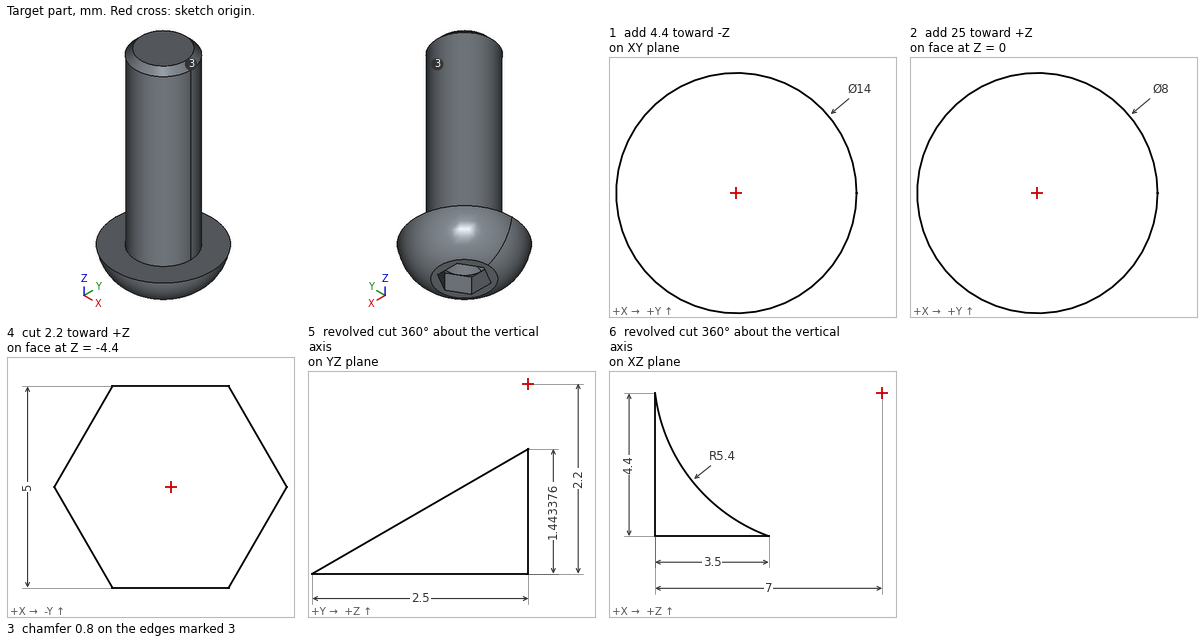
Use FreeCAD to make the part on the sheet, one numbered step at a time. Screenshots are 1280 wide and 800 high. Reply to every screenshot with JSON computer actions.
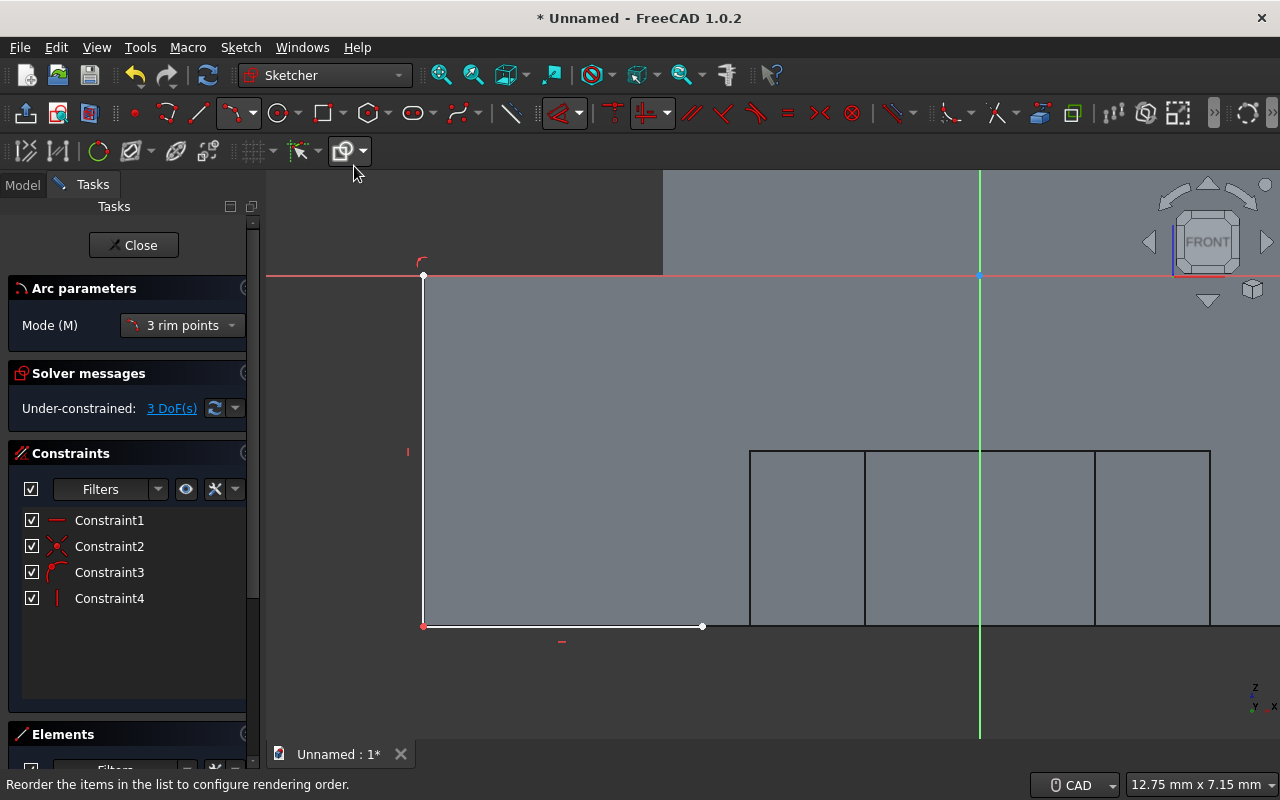
{"action": "left_click", "coordinate": [423, 276]}
{"action": "left_click", "coordinate": [702, 627]}
{"action": "left_click", "coordinate": [513, 490]}
{"action": "key", "text": "Escape"}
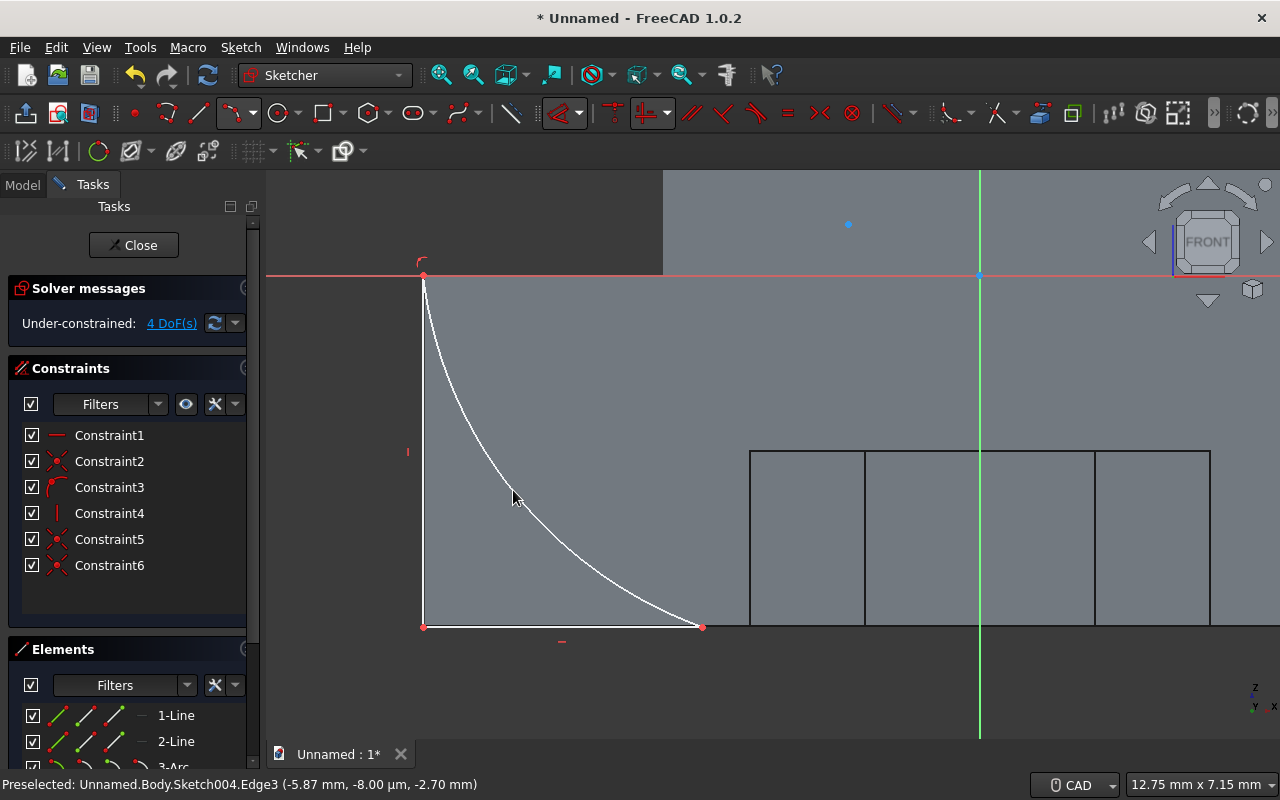
{"action": "left_click", "coordinate": [463, 411]}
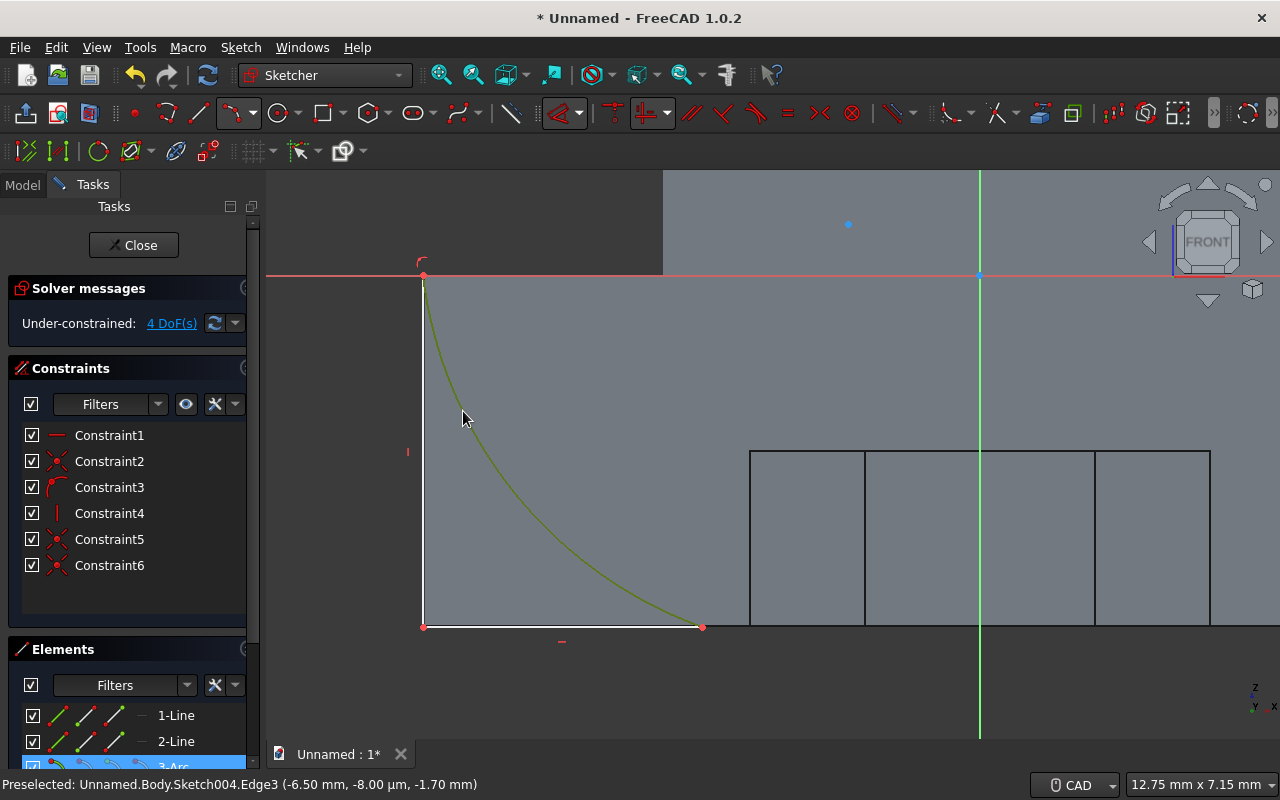
{"action": "key", "text": "k r"}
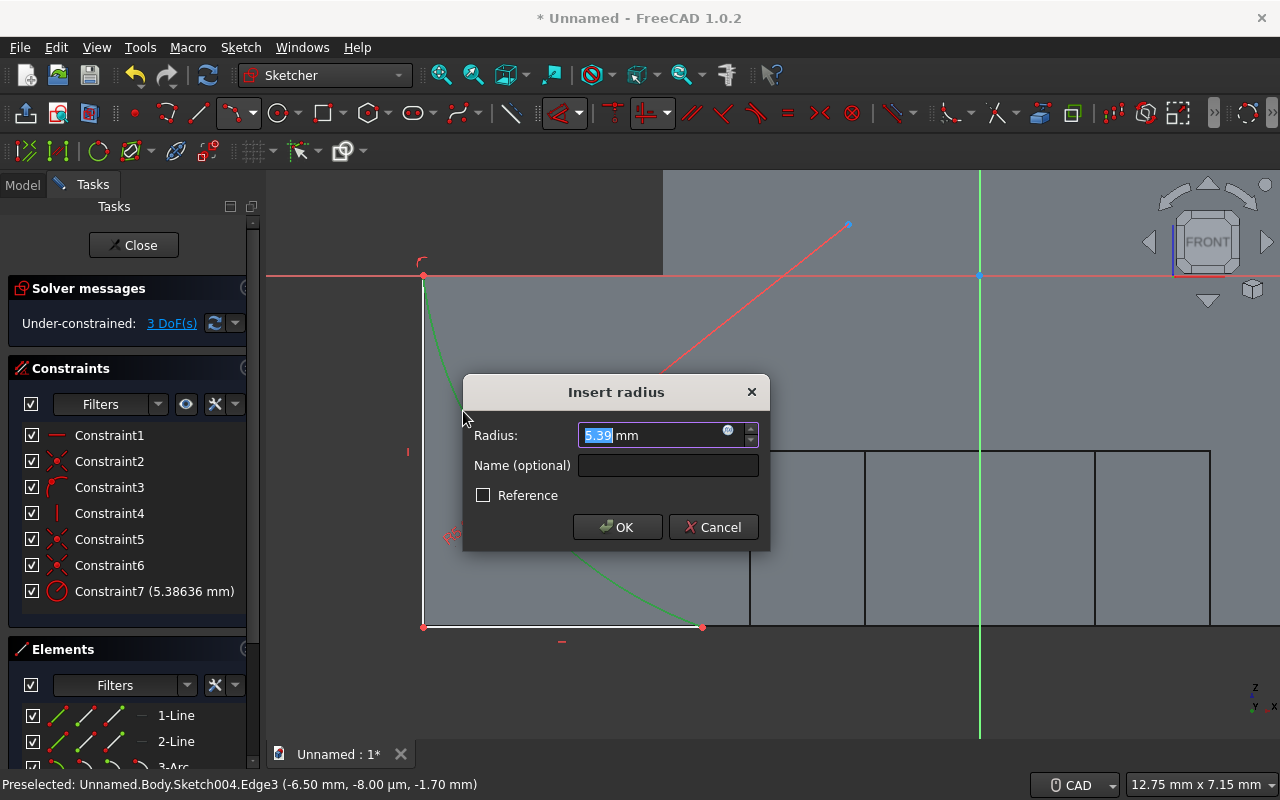
{"action": "type", "text": "5.4"}
{"action": "key", "text": "Return"}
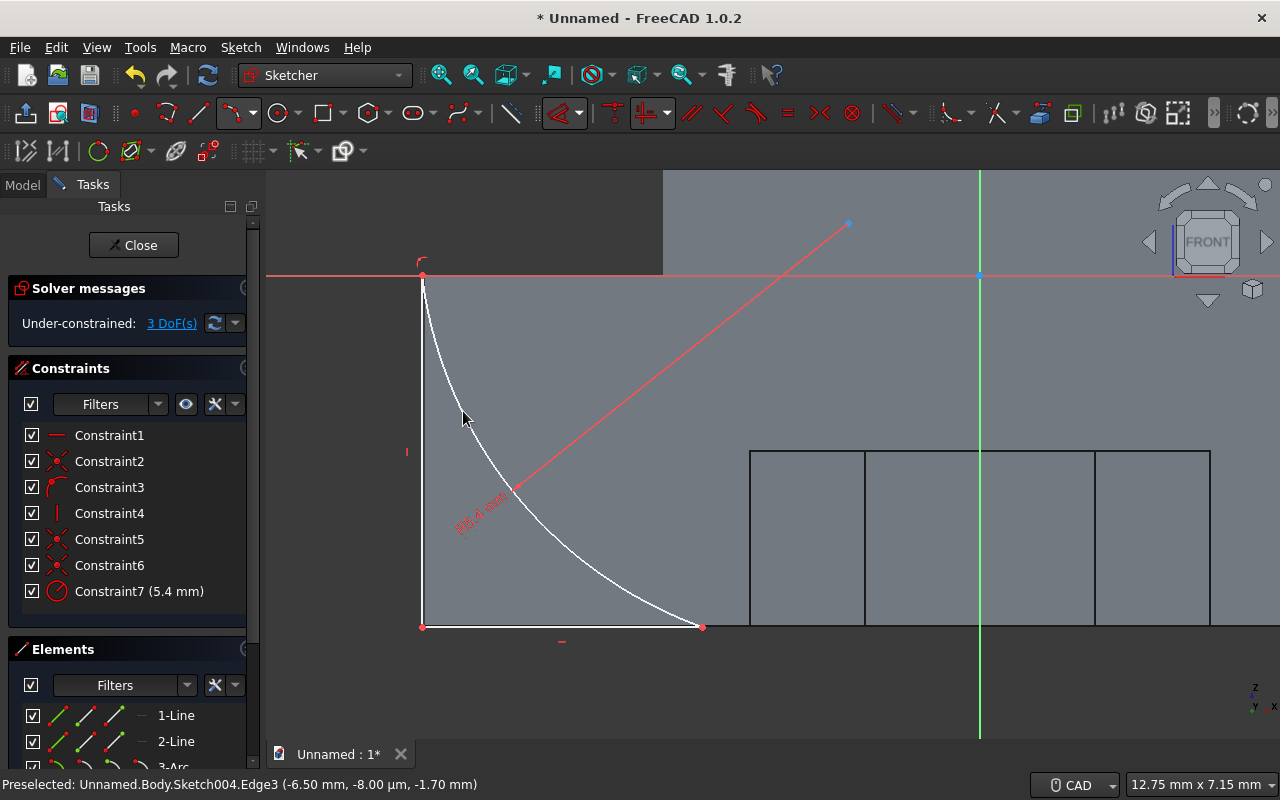
{"action": "left_click", "coordinate": [422, 627]}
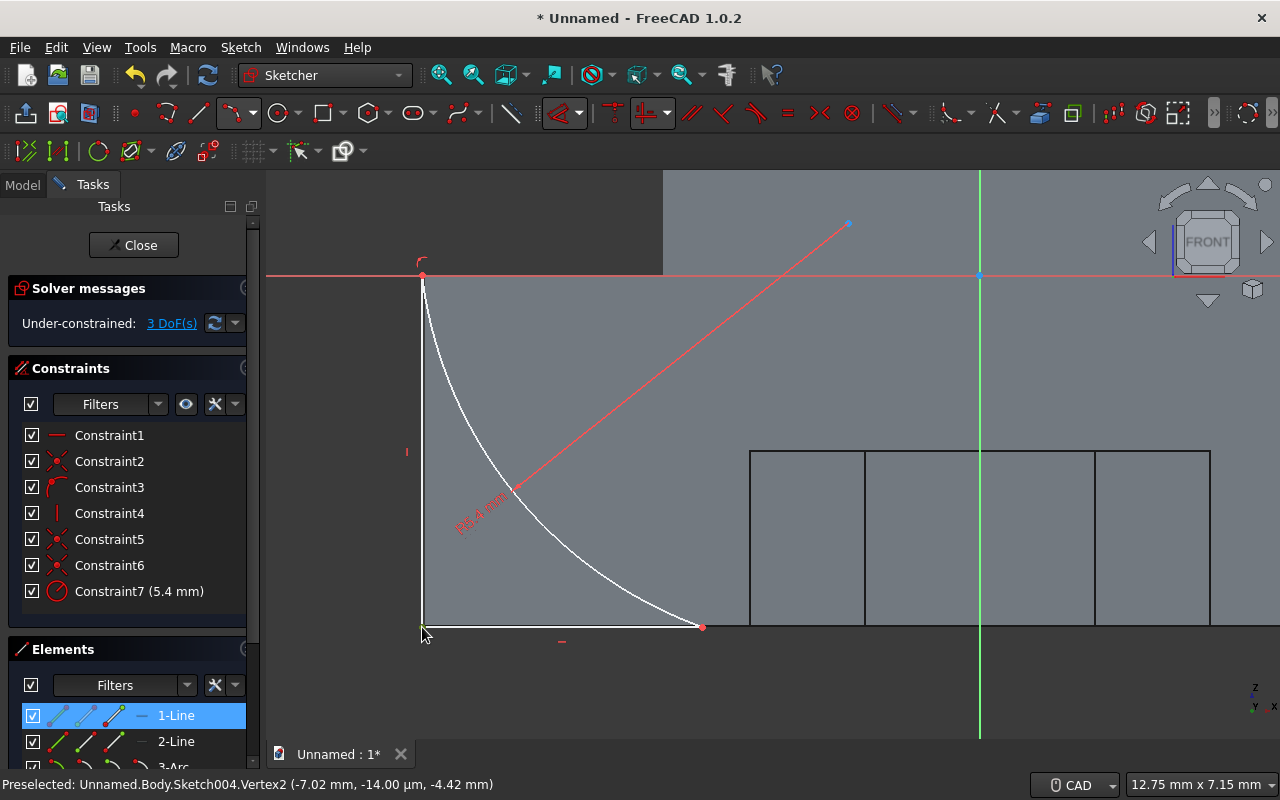
{"action": "key", "text": "l"}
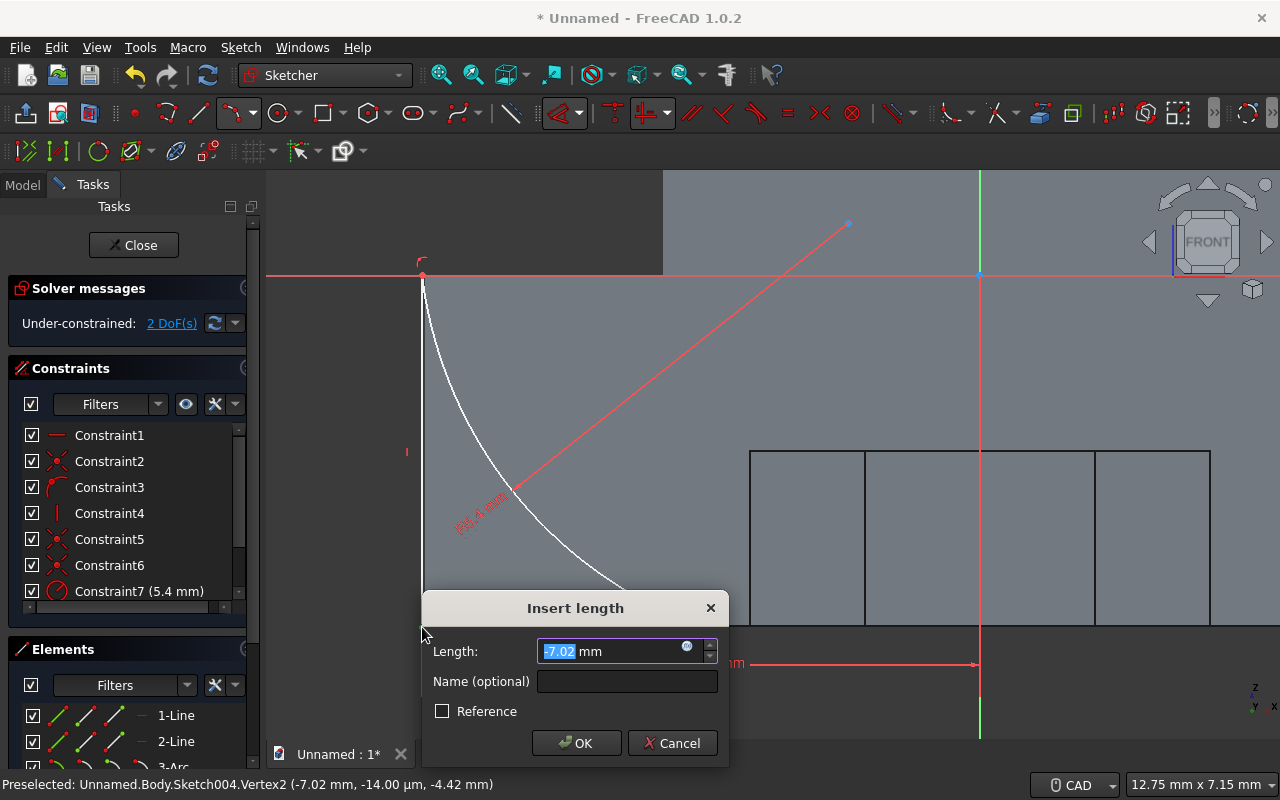
{"action": "type", "text": "-7"}
{"action": "key", "text": "Return"}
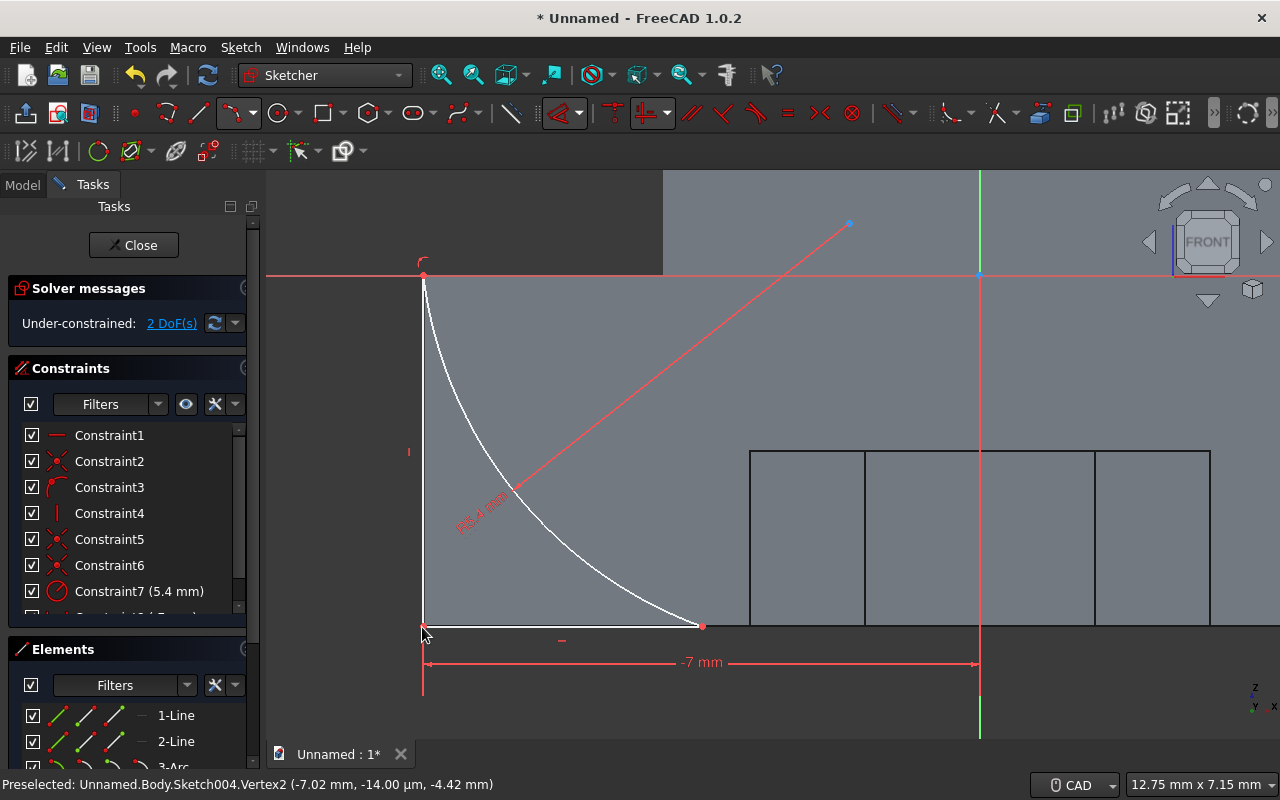
{"action": "left_click", "coordinate": [618, 627]}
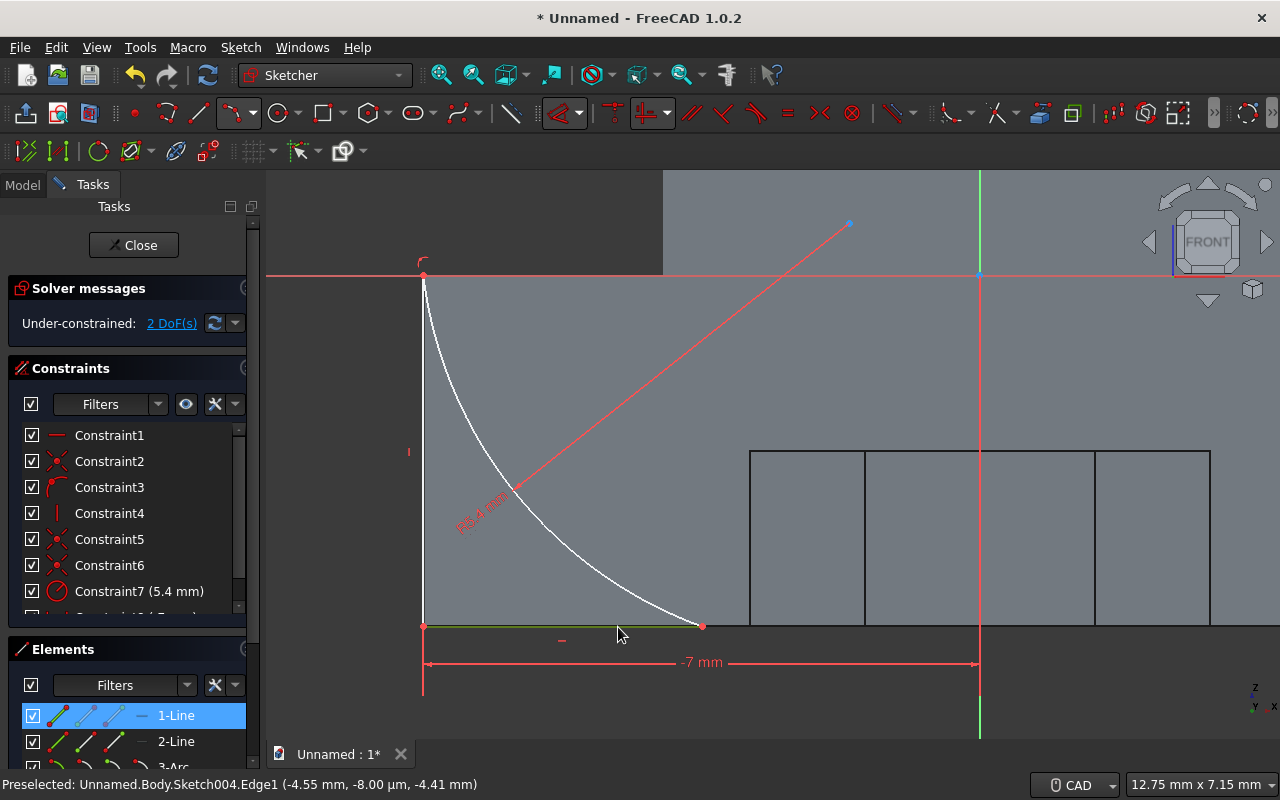
{"action": "left_click", "coordinate": [582, 114]}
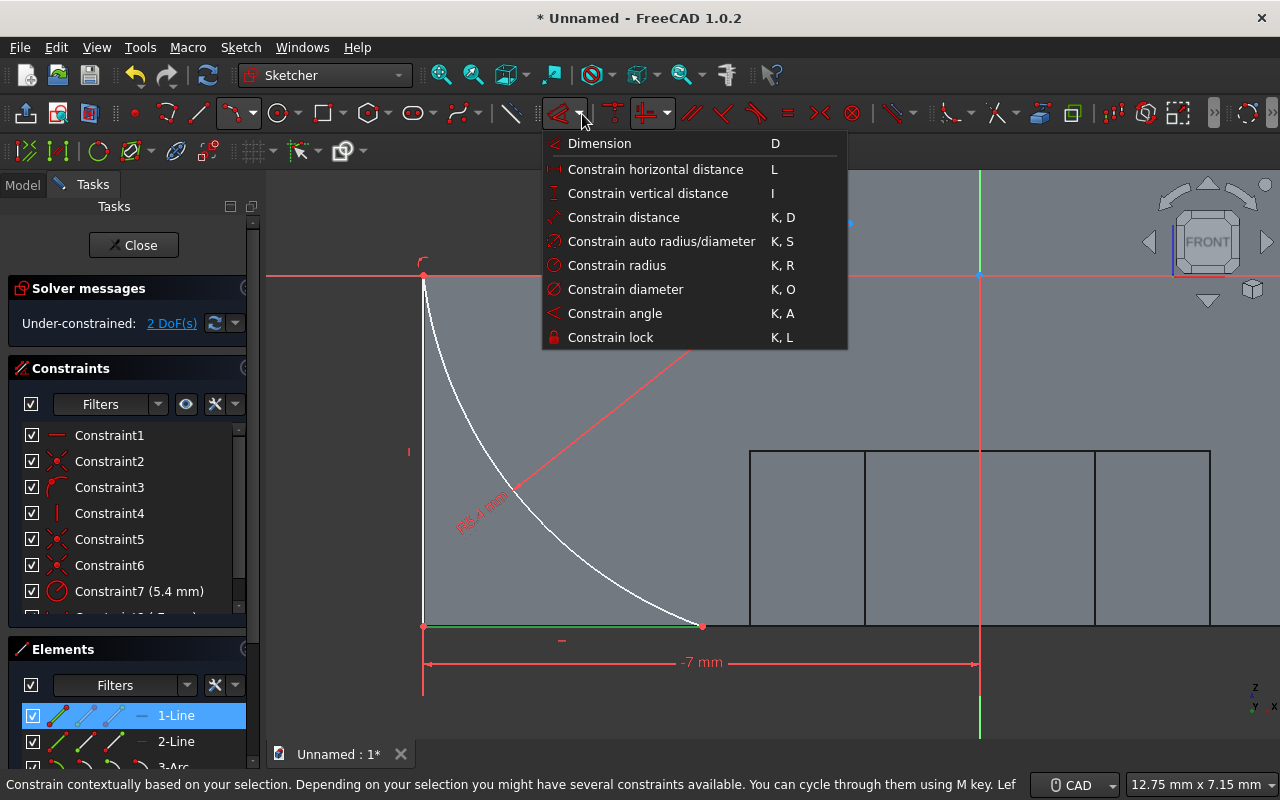
{"action": "left_click", "coordinate": [695, 169]}